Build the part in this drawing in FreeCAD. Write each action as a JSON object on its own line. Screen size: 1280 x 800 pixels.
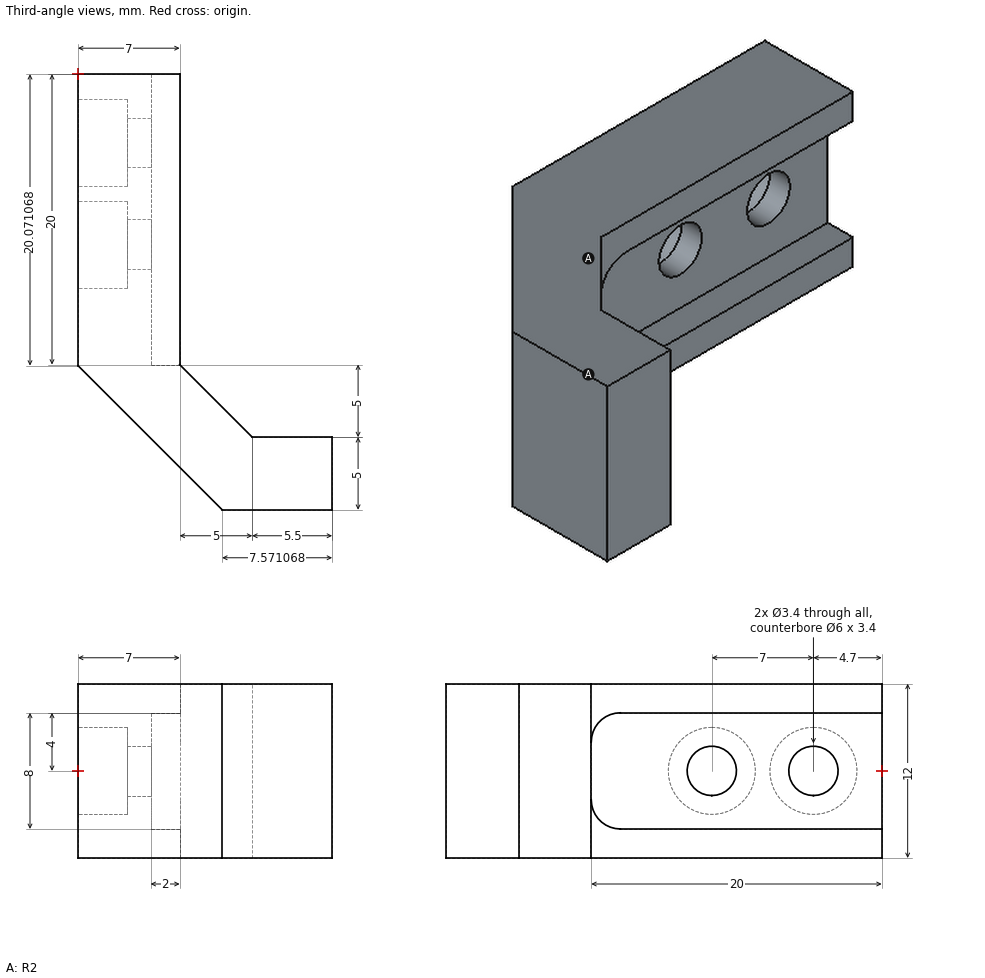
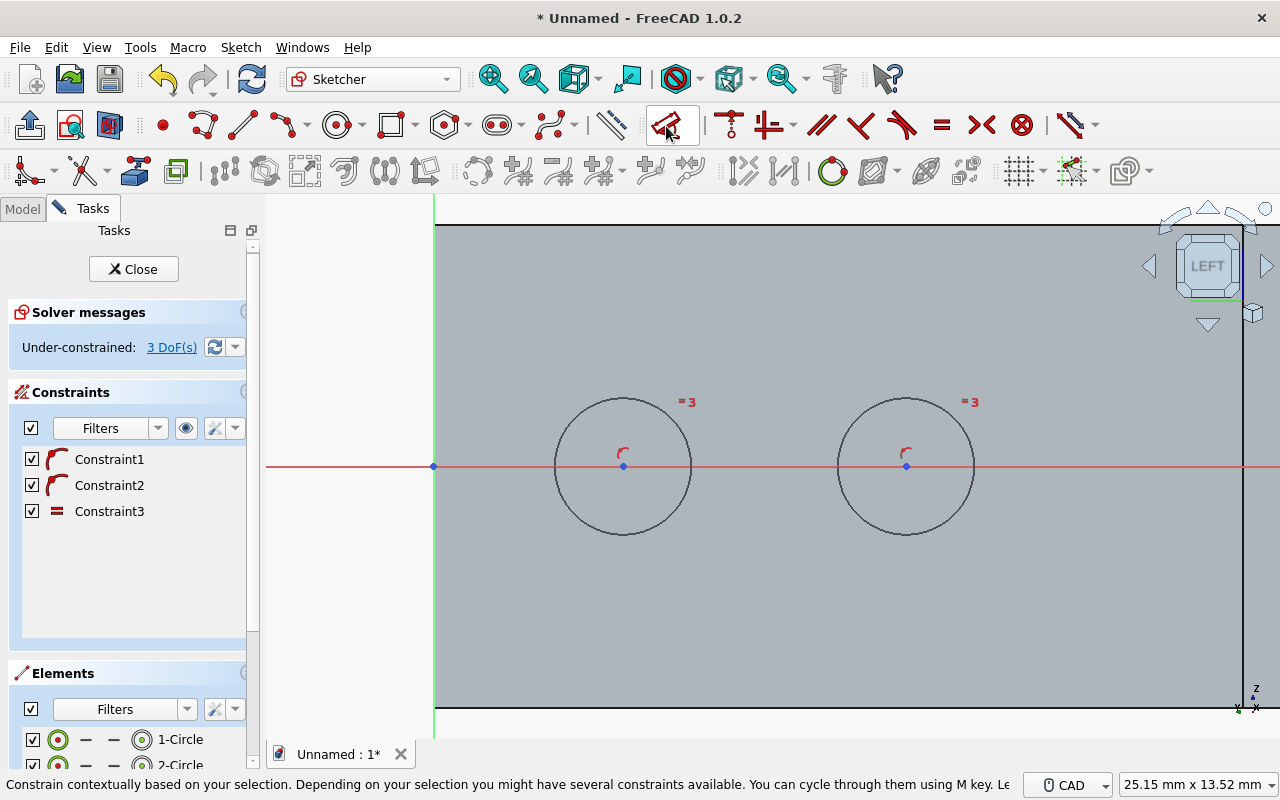
{"action": "left_click", "coordinate": [671, 418]}
{"action": "left_click", "coordinate": [694, 395]}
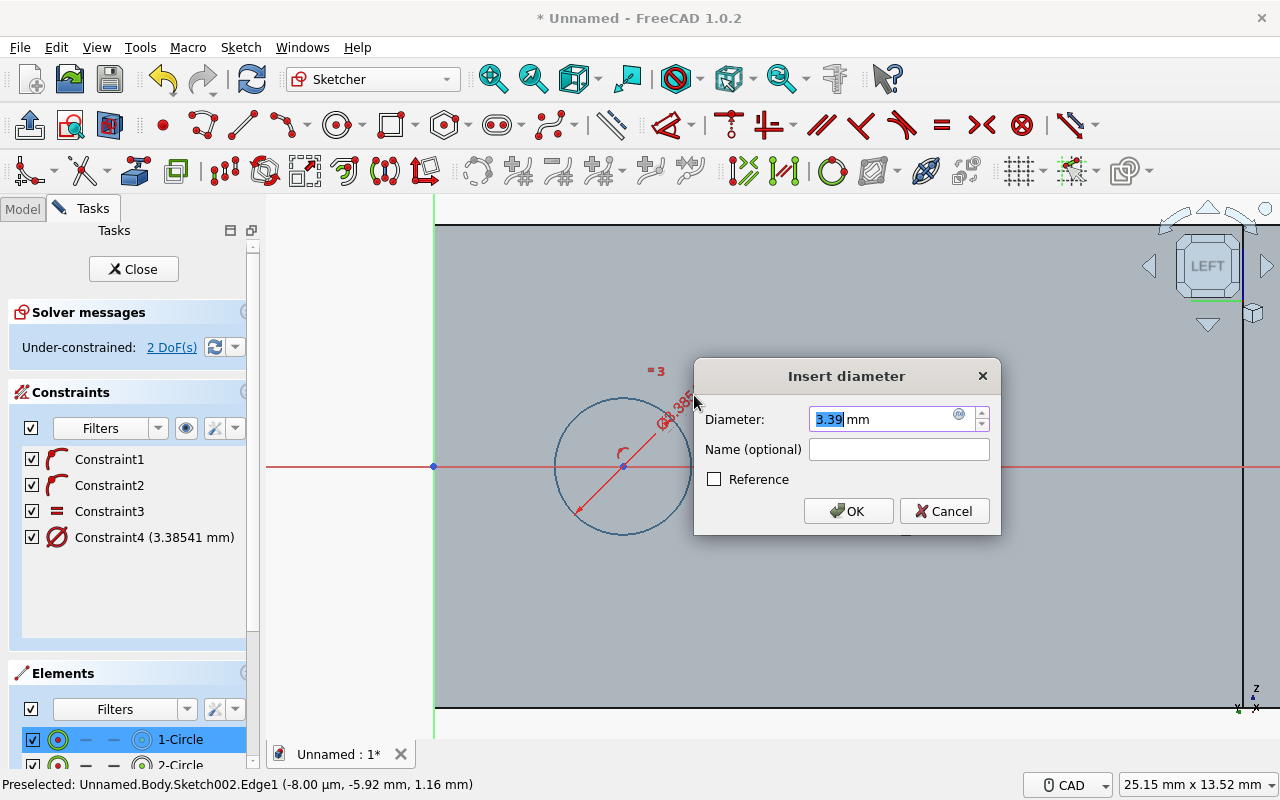
{"action": "type", "text": "3.4"}
{"action": "key", "text": "Return"}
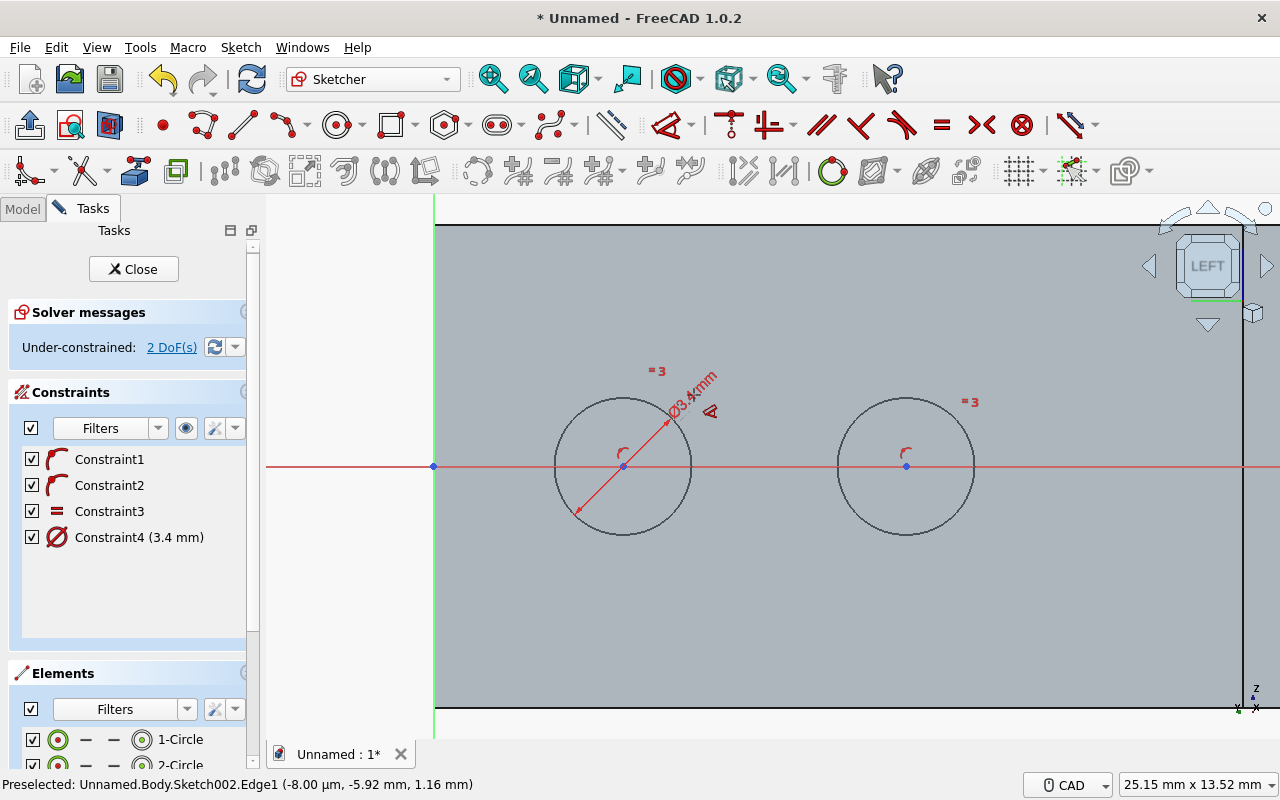
{"action": "left_click", "coordinate": [623, 466]}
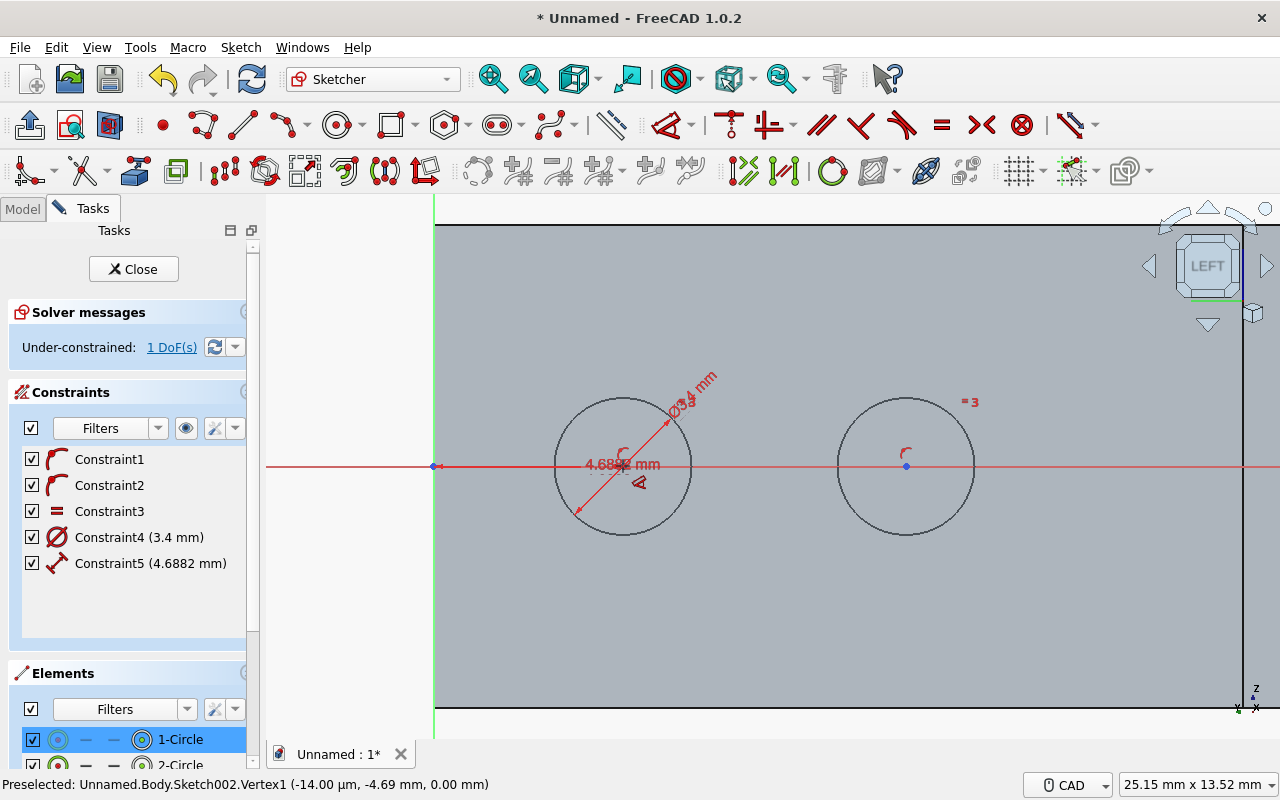
{"action": "left_click", "coordinate": [906, 466]}
{"action": "left_click", "coordinate": [765, 500]}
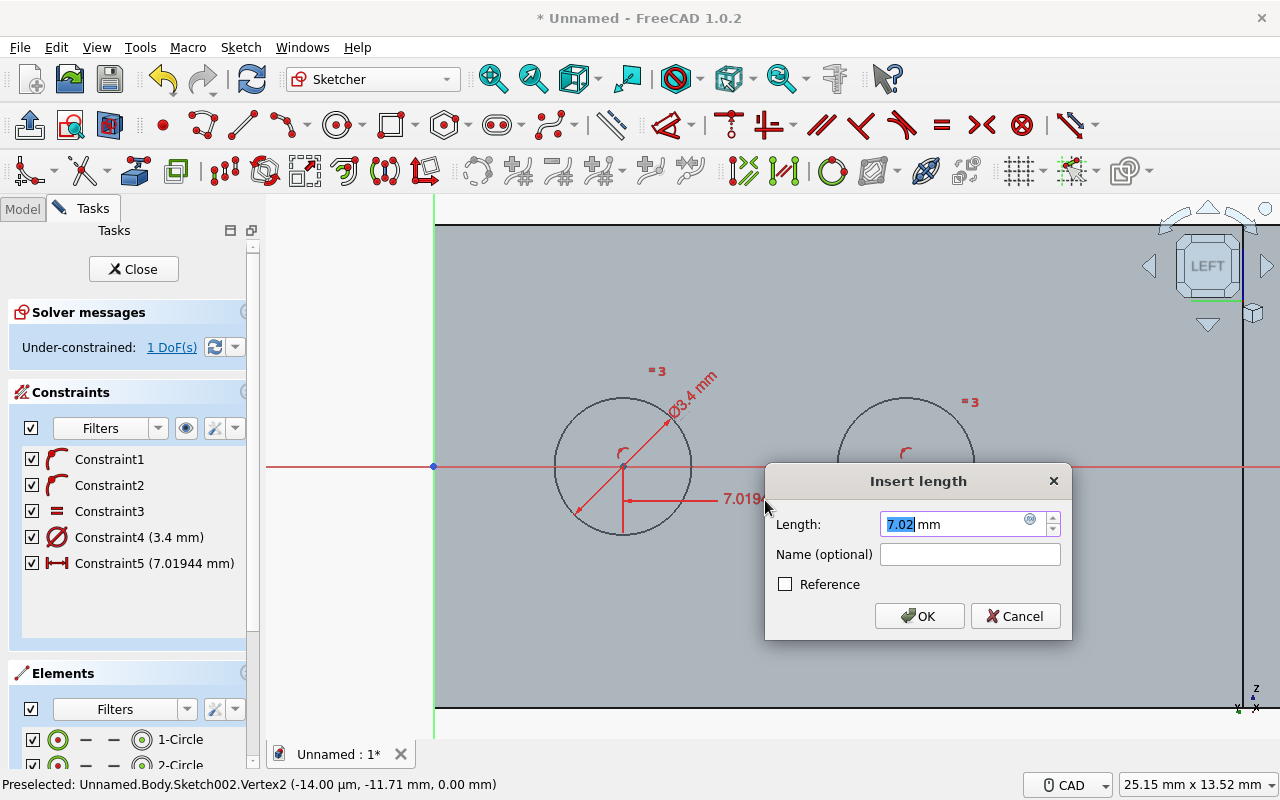
{"action": "type", "text": "7"}
{"action": "key", "text": "Return"}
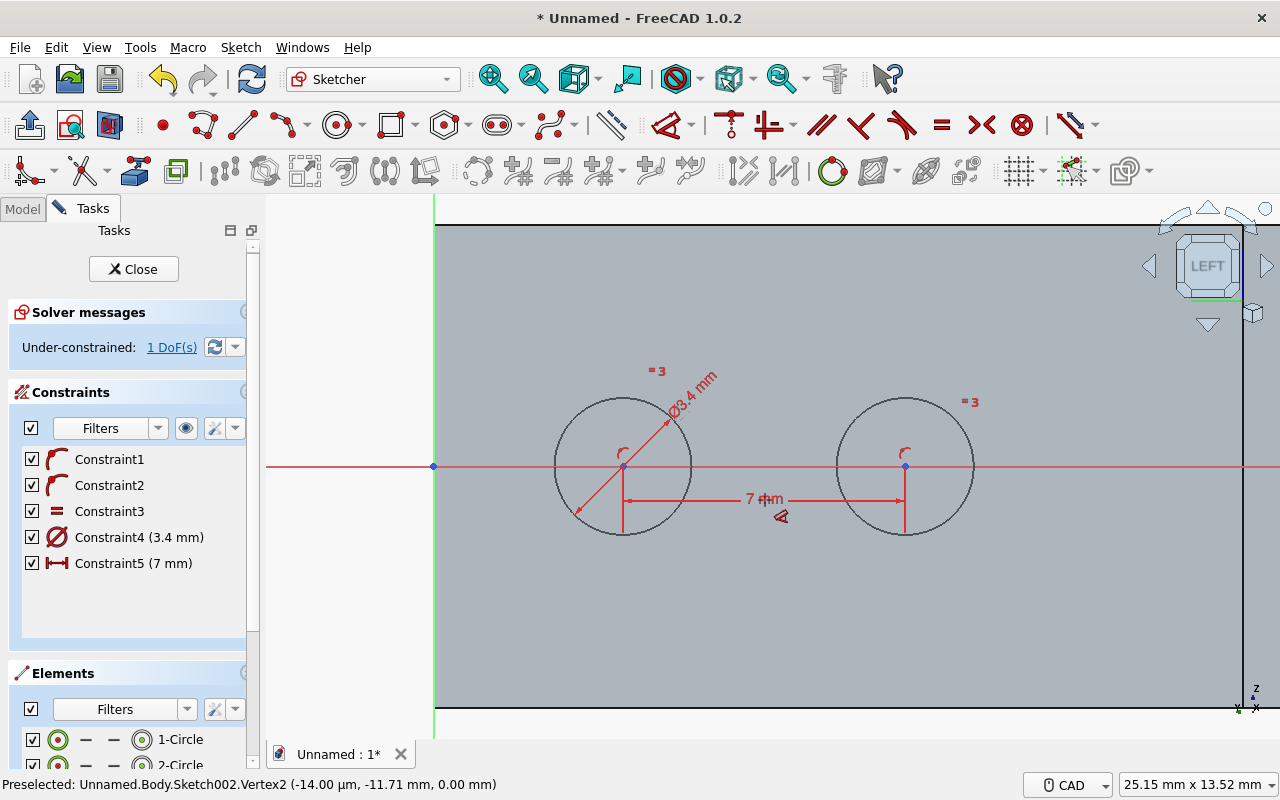
{"action": "left_click", "coordinate": [623, 466]}
{"action": "left_click", "coordinate": [528, 500]}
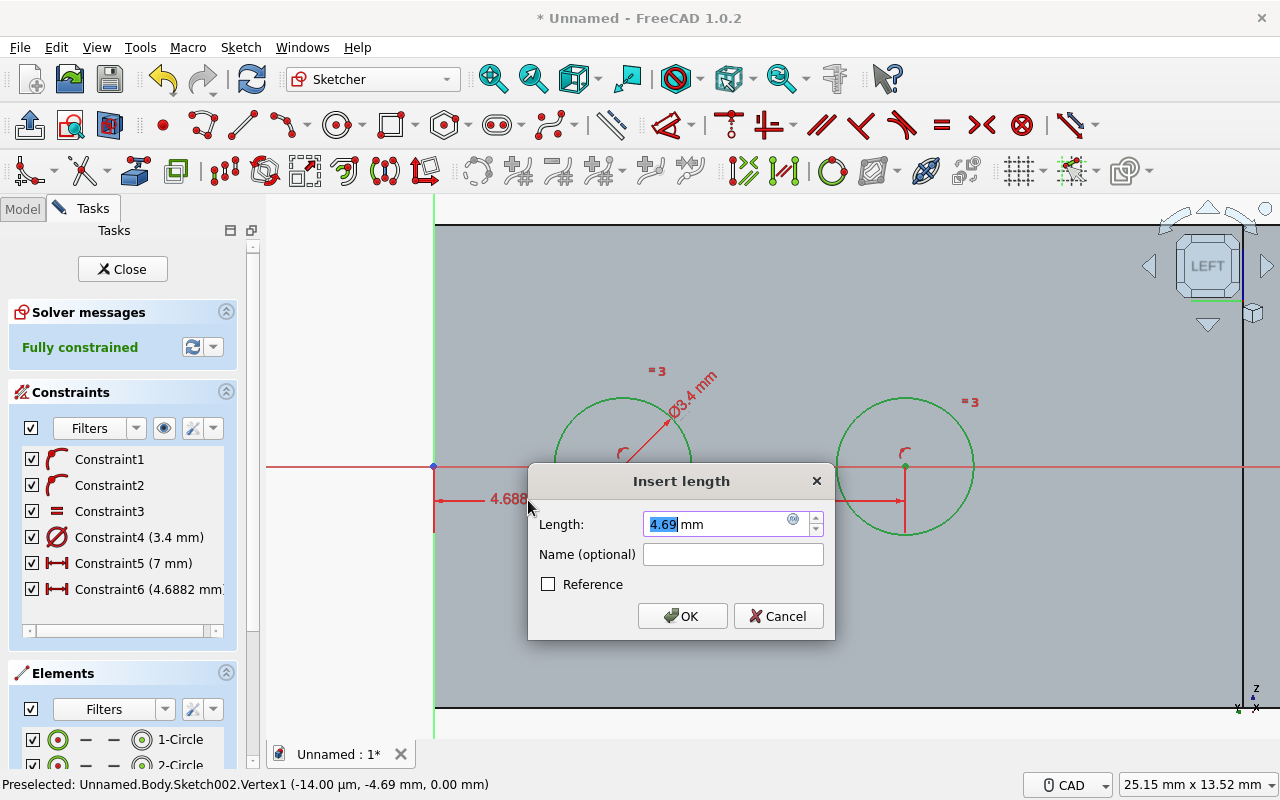
{"action": "type", "text": "4.7"}
{"action": "key", "text": "Return"}
{"action": "key", "text": "Escape"}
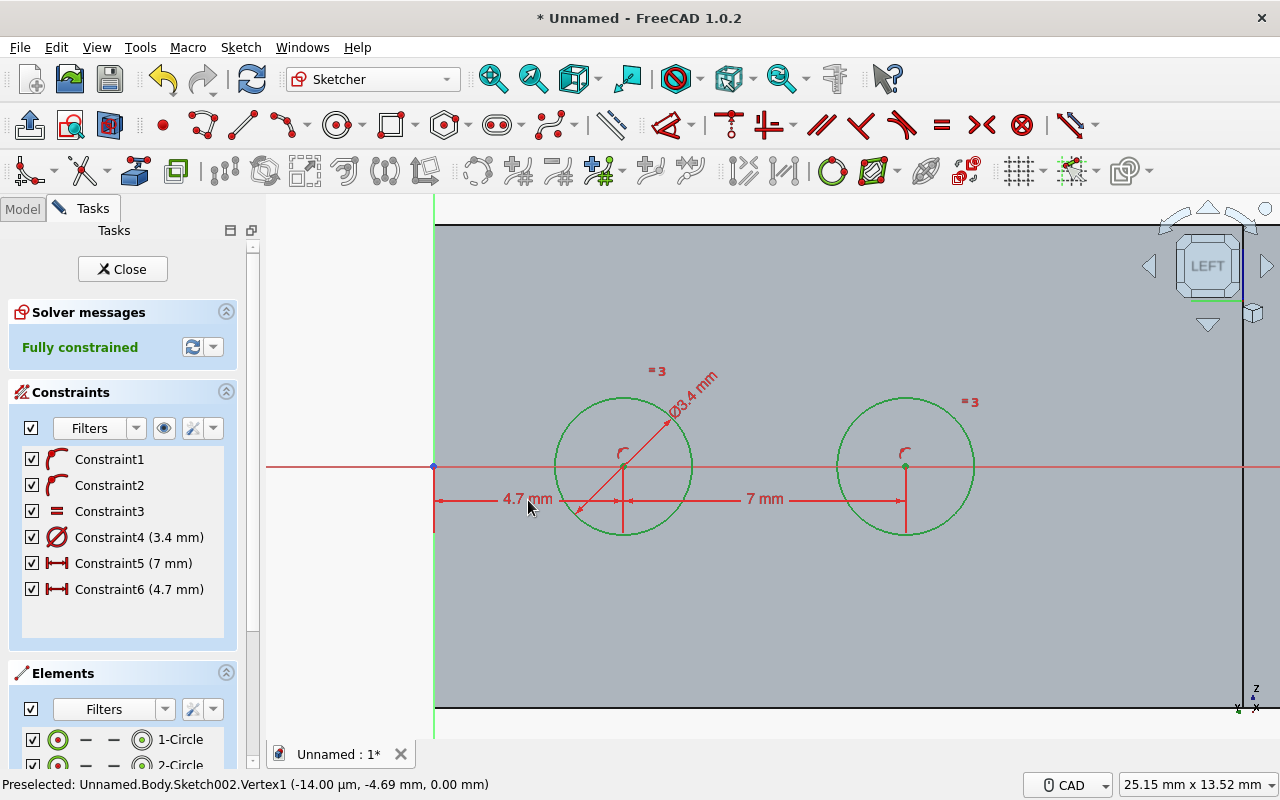
{"action": "left_click", "coordinate": [123, 269]}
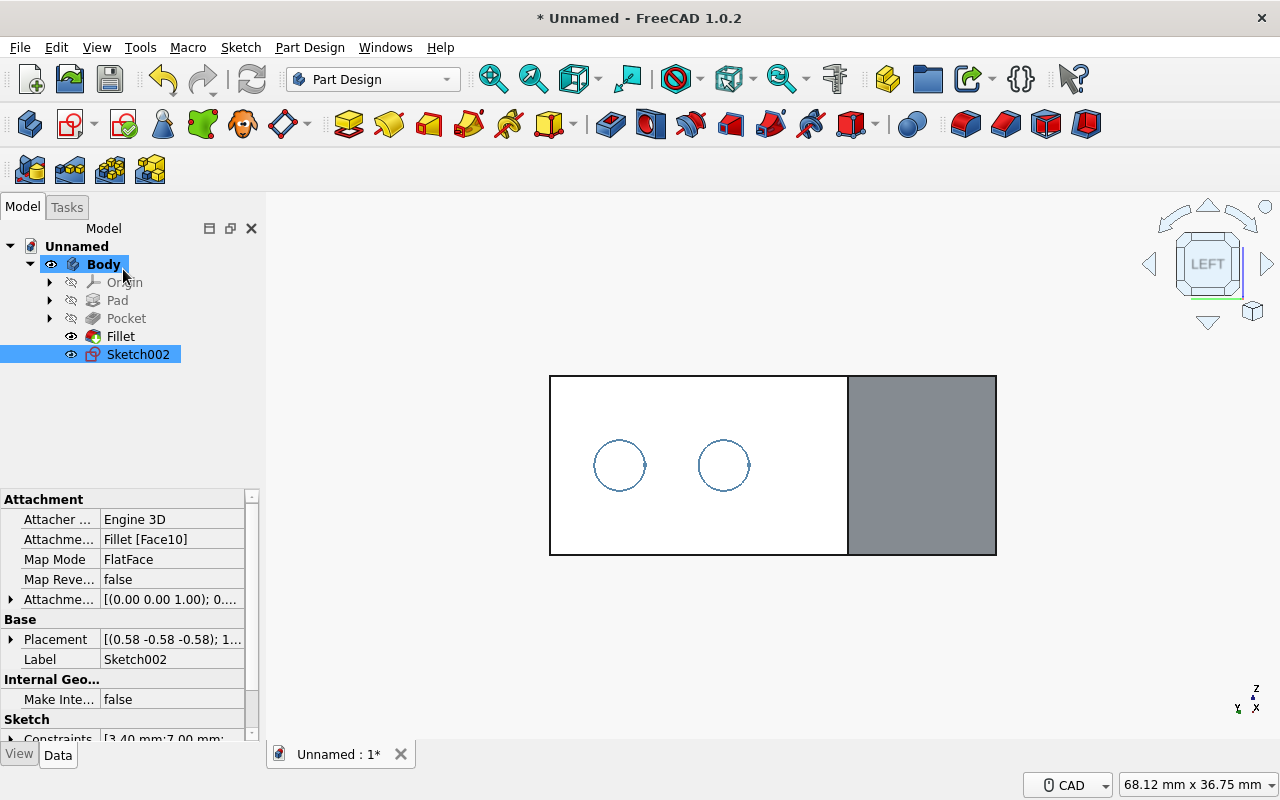
{"action": "left_click", "coordinate": [652, 124]}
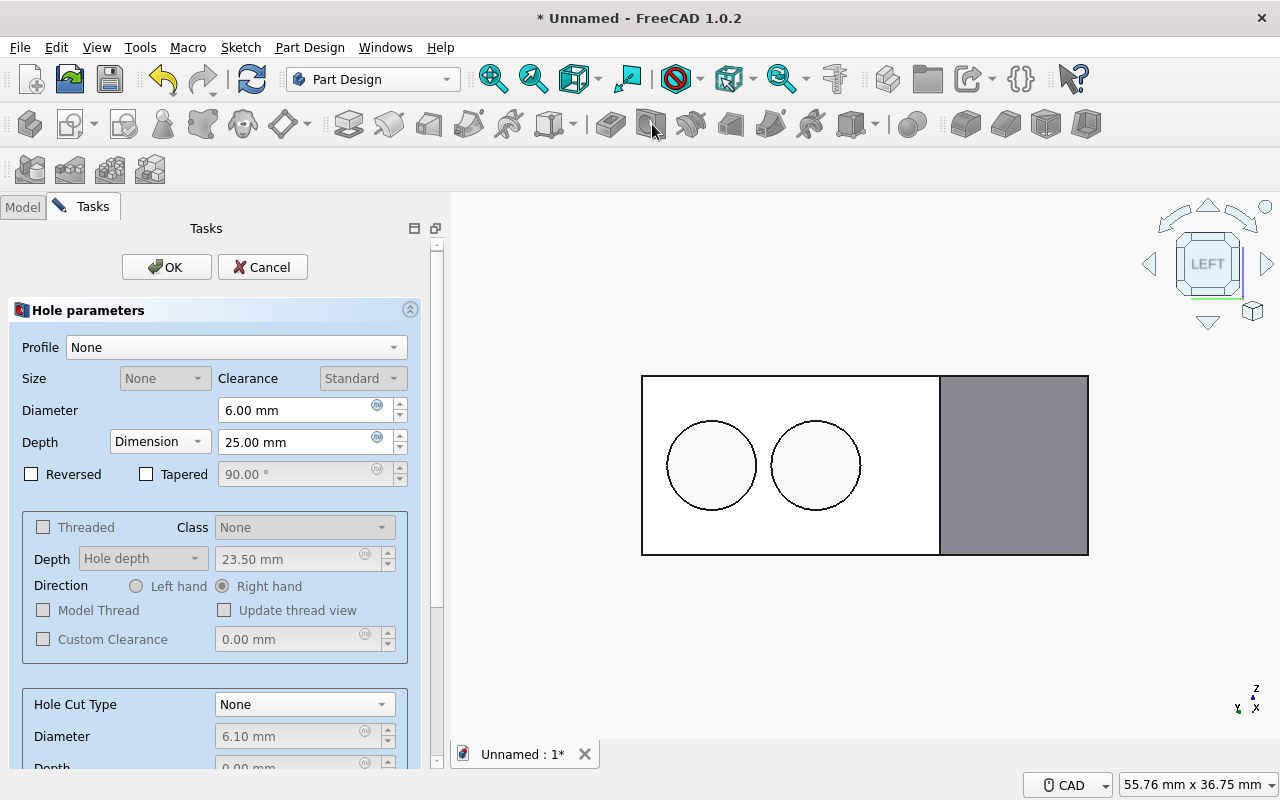
{"action": "triple_click", "coordinate": [305, 410]}